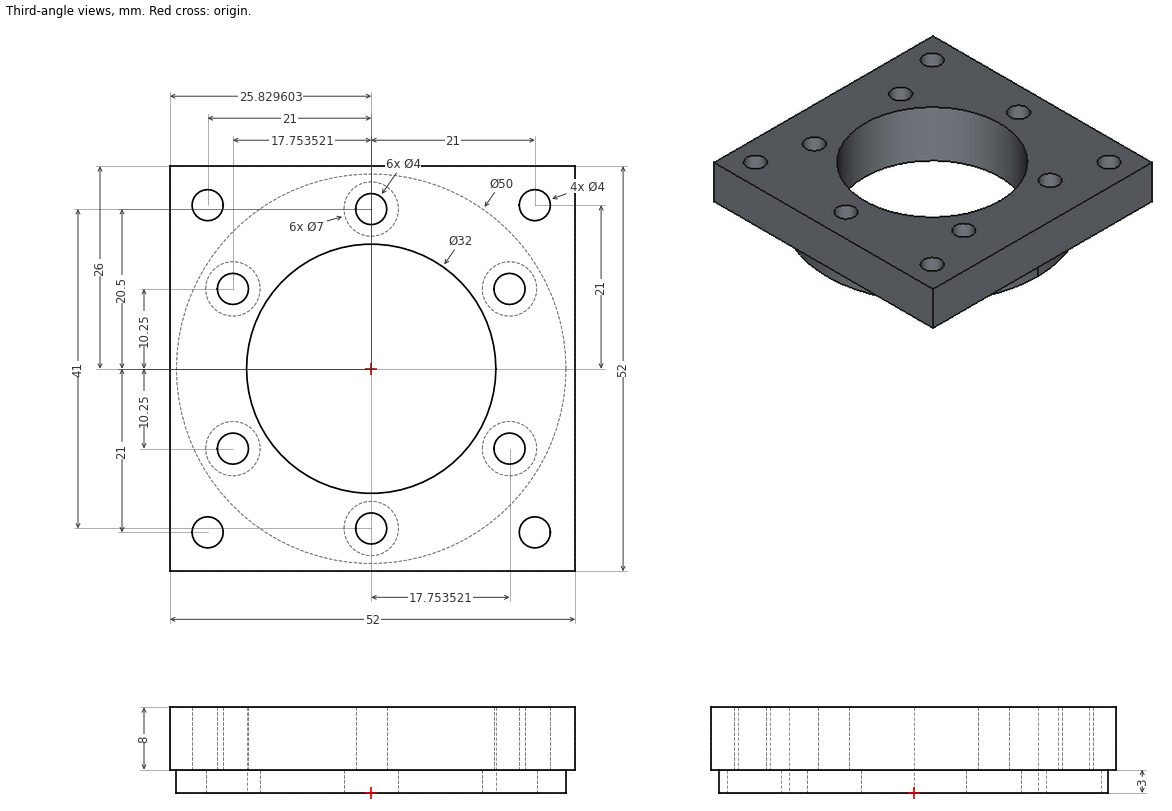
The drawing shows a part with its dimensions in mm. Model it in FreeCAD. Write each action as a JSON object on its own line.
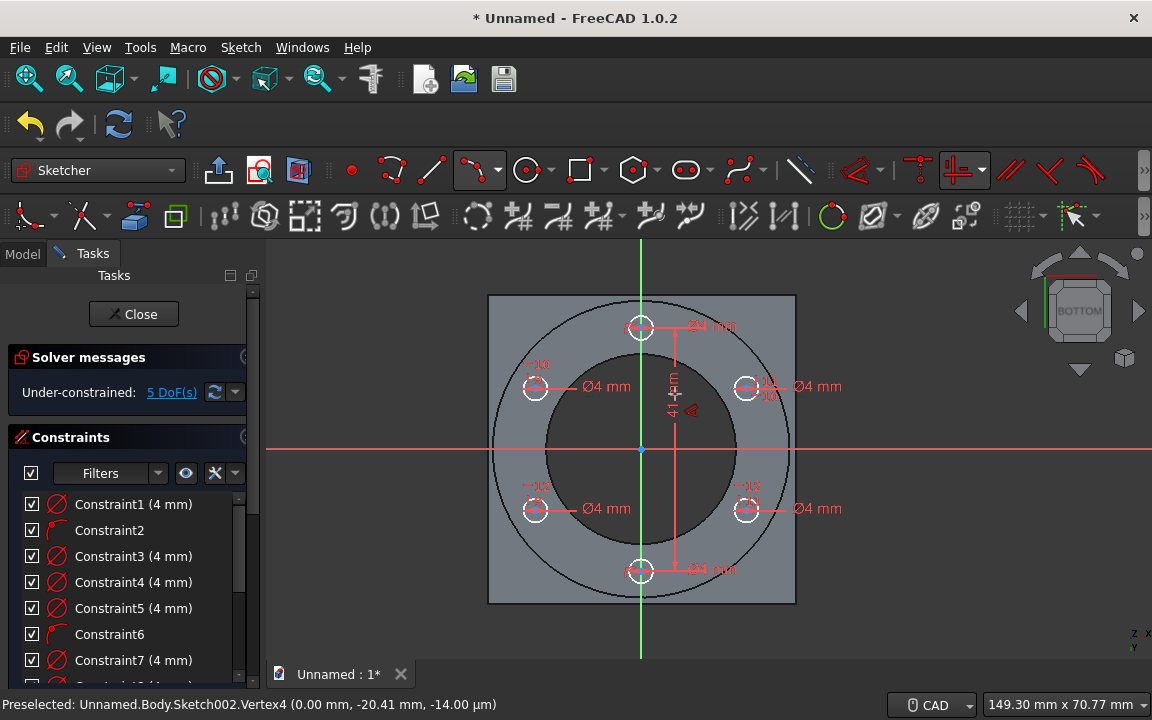
{"action": "left_click", "coordinate": [641, 571]}
{"action": "left_click", "coordinate": [675, 510]}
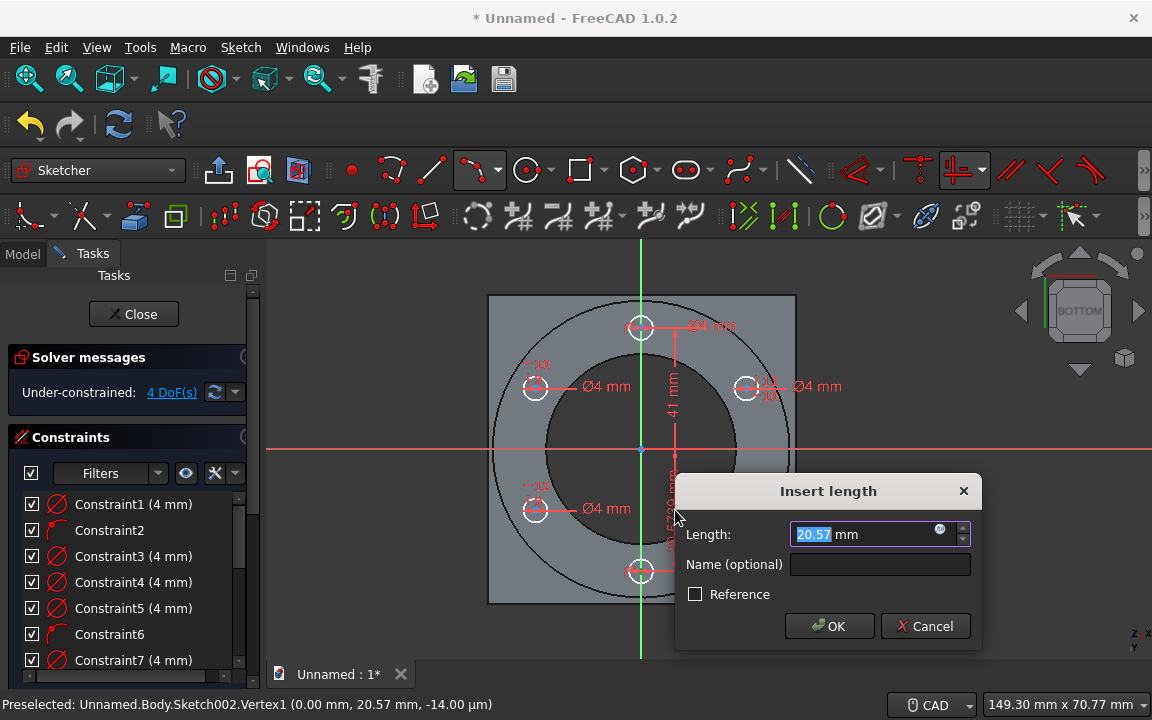
{"action": "type", "text": "20.5"}
{"action": "key", "text": "Return"}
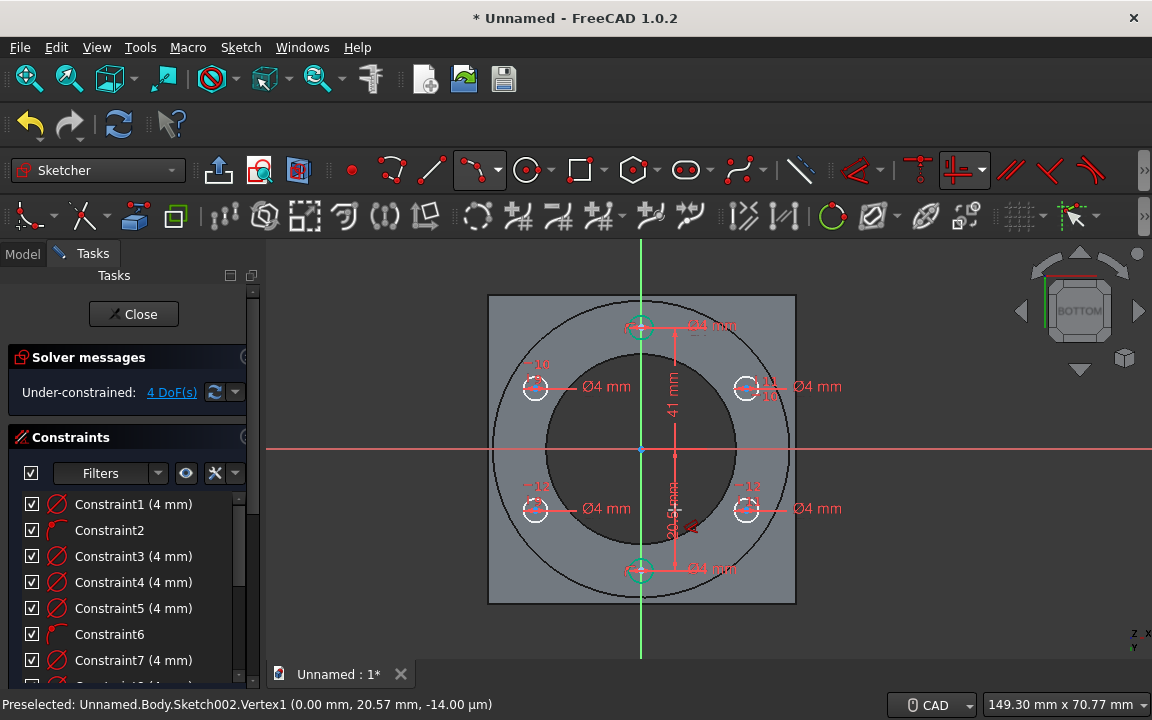
{"action": "left_click", "coordinate": [536, 511]}
{"action": "left_click", "coordinate": [502, 480]}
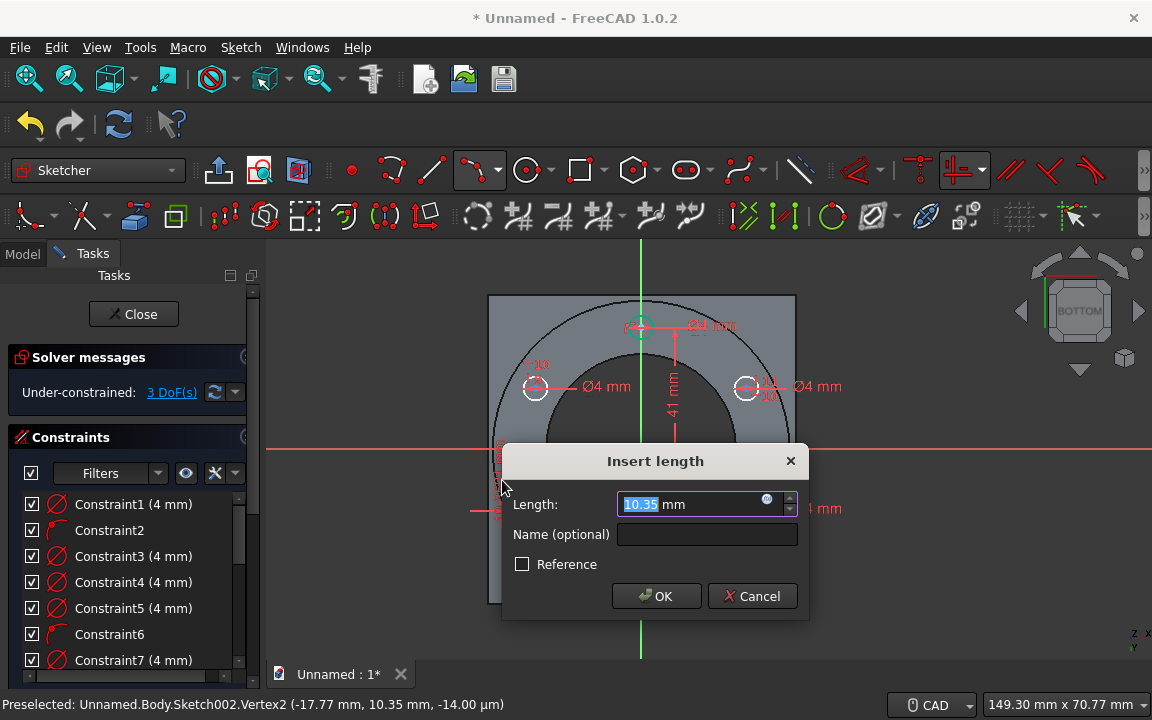
{"action": "type", "text": "10.25"}
{"action": "key", "text": "Return"}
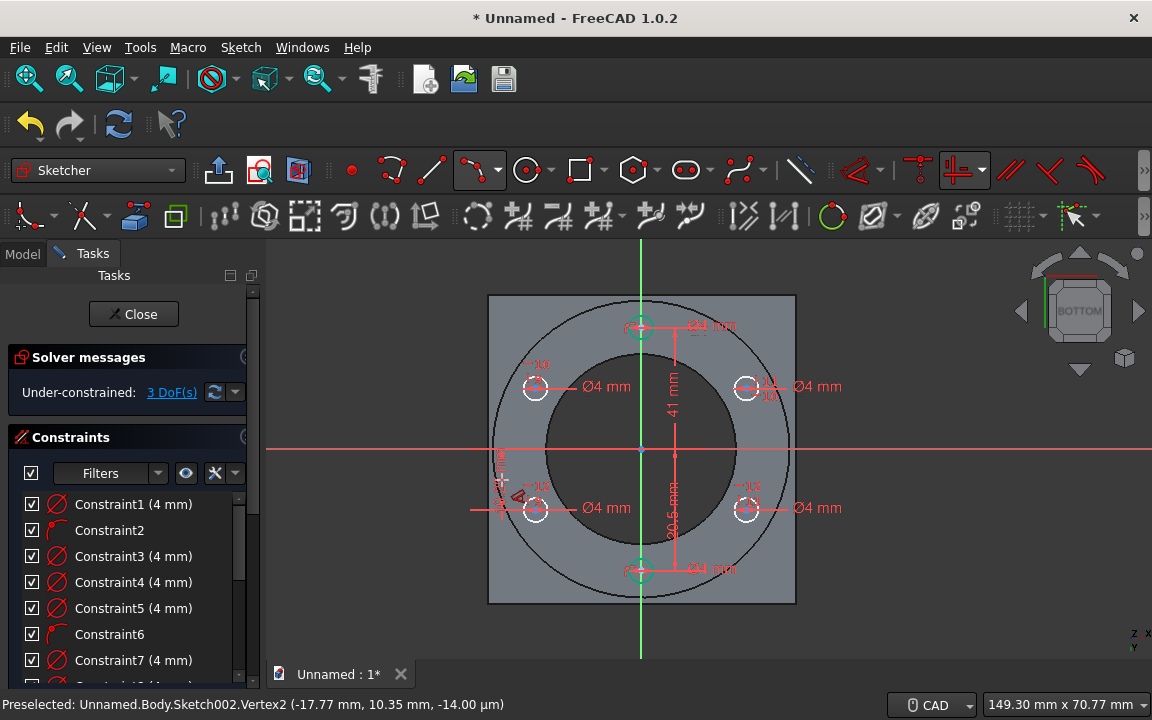
{"action": "left_click", "coordinate": [536, 389]}
{"action": "left_click", "coordinate": [502, 419]}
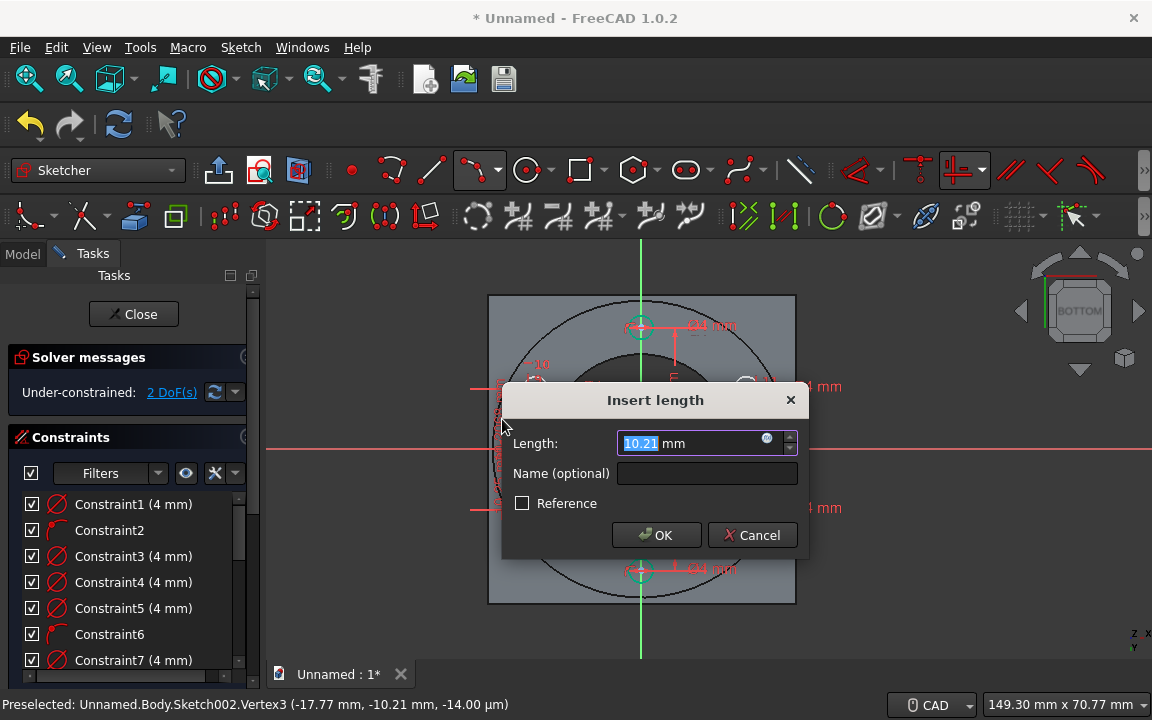
{"action": "type", "text": "10.25"}
{"action": "key", "text": "Return"}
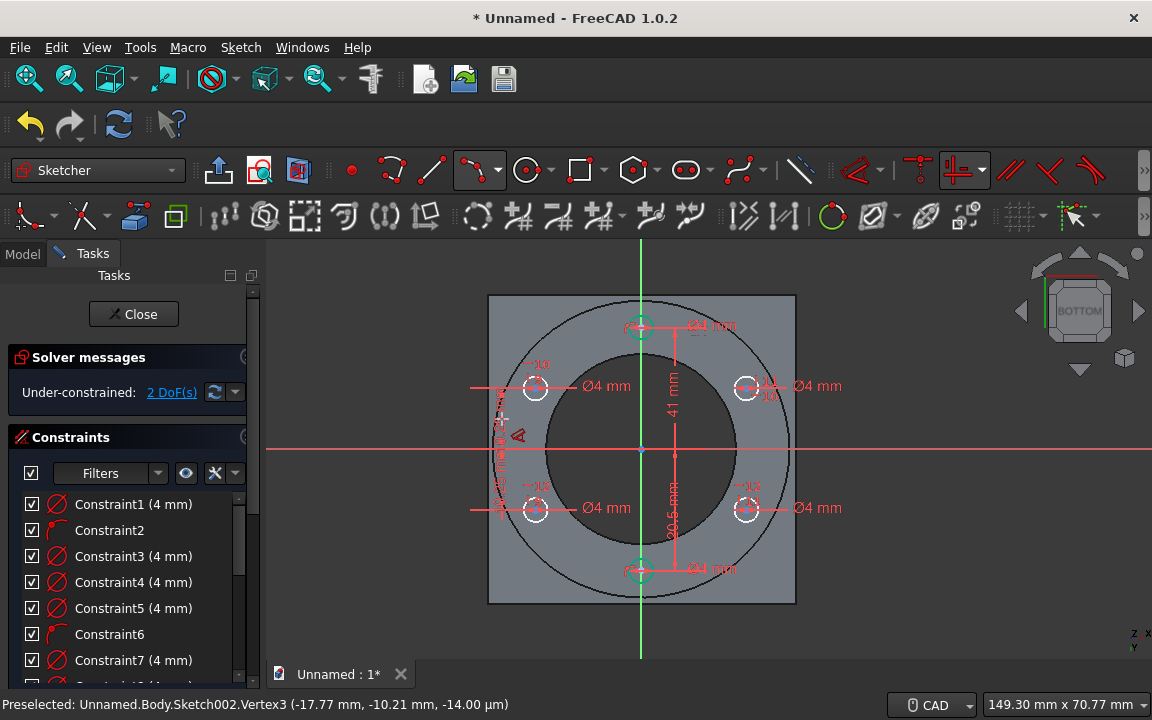
{"action": "left_click", "coordinate": [536, 510]}
{"action": "left_click", "coordinate": [588, 544]}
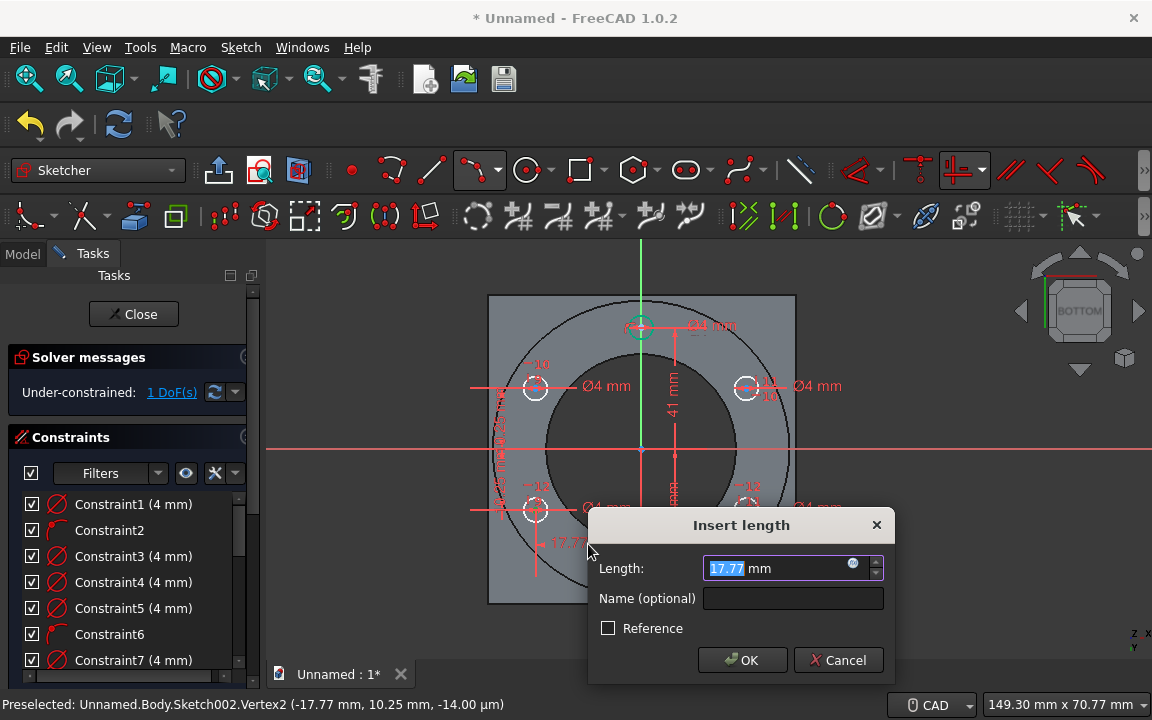
{"action": "type", "text": "17.753521"}
{"action": "key", "text": "Return"}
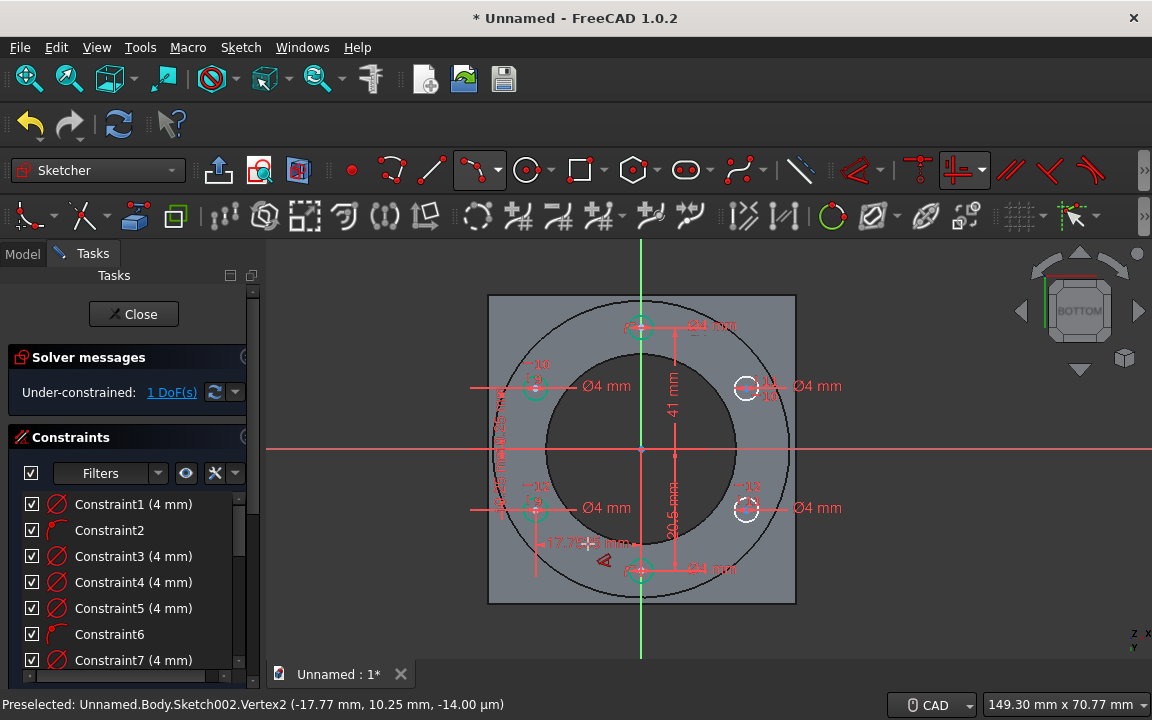
{"action": "left_click", "coordinate": [746, 388]}
{"action": "left_click", "coordinate": [694, 354]}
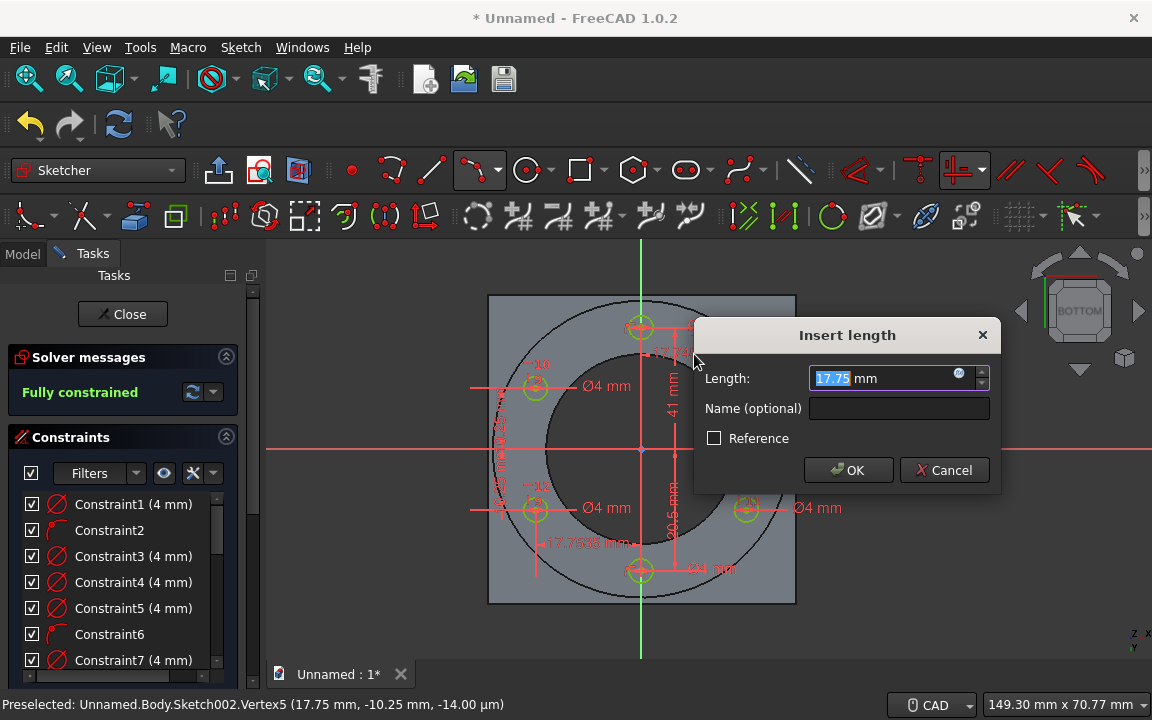
{"action": "type", "text": "17.753521"}
{"action": "key", "text": "Return"}
{"action": "key", "text": "Escape"}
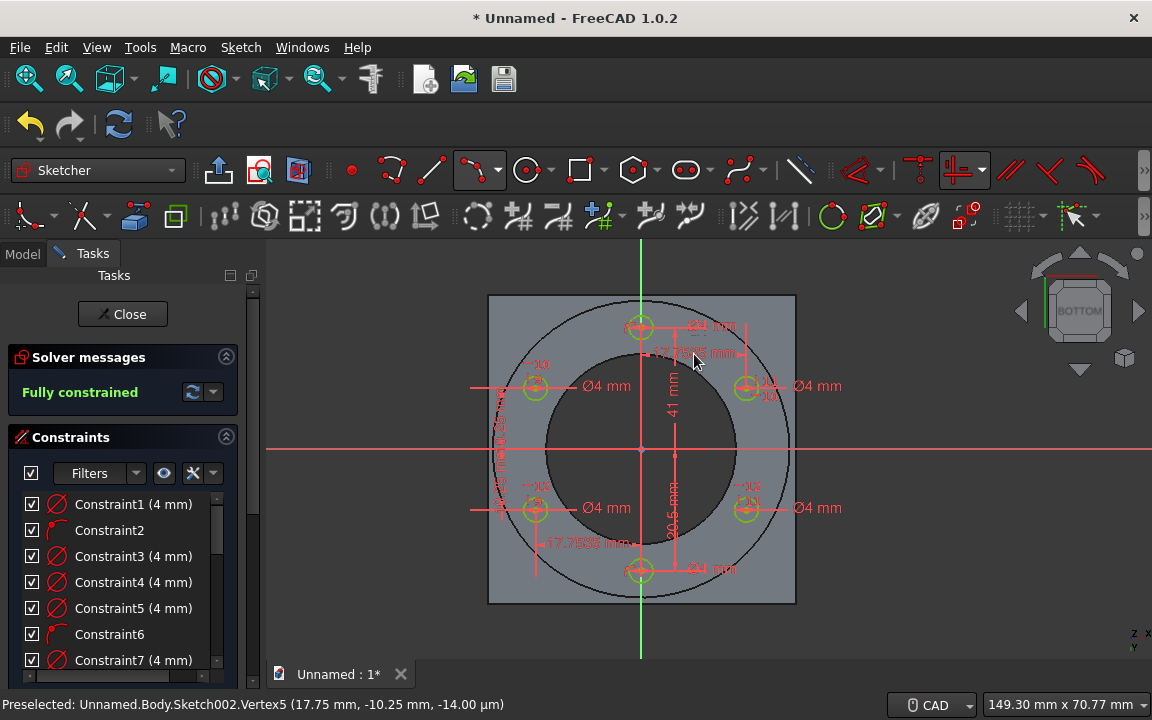
{"action": "left_click", "coordinate": [123, 314]}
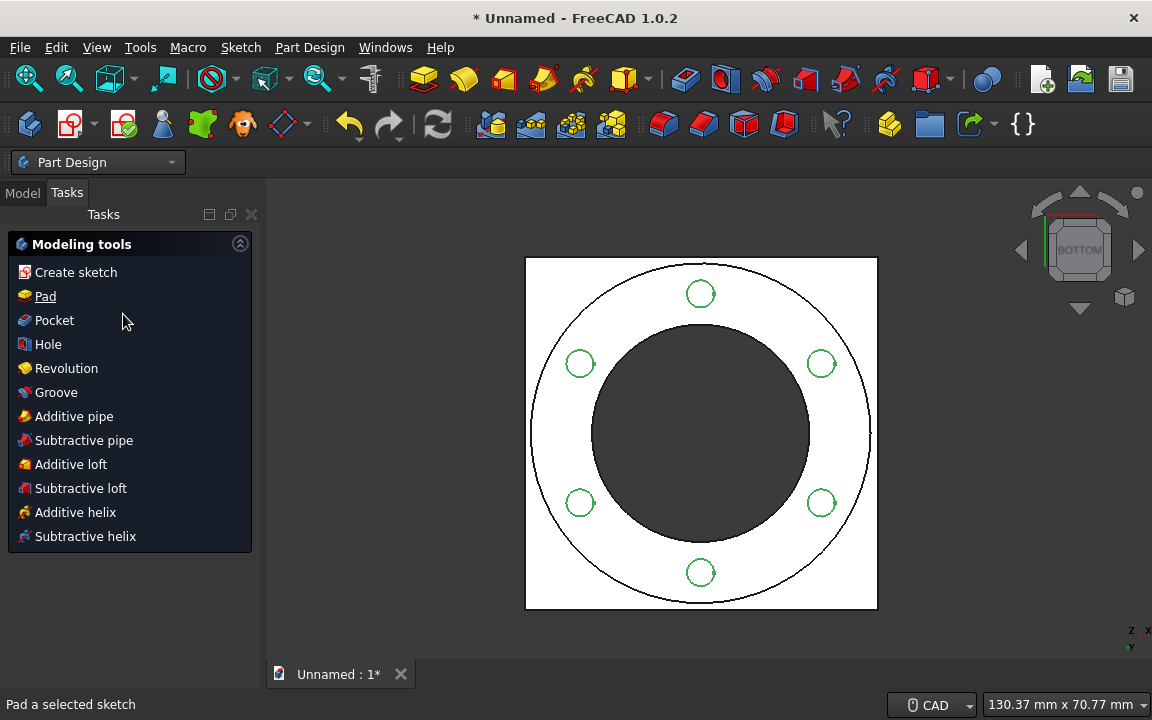
{"action": "left_click", "coordinate": [686, 80]}